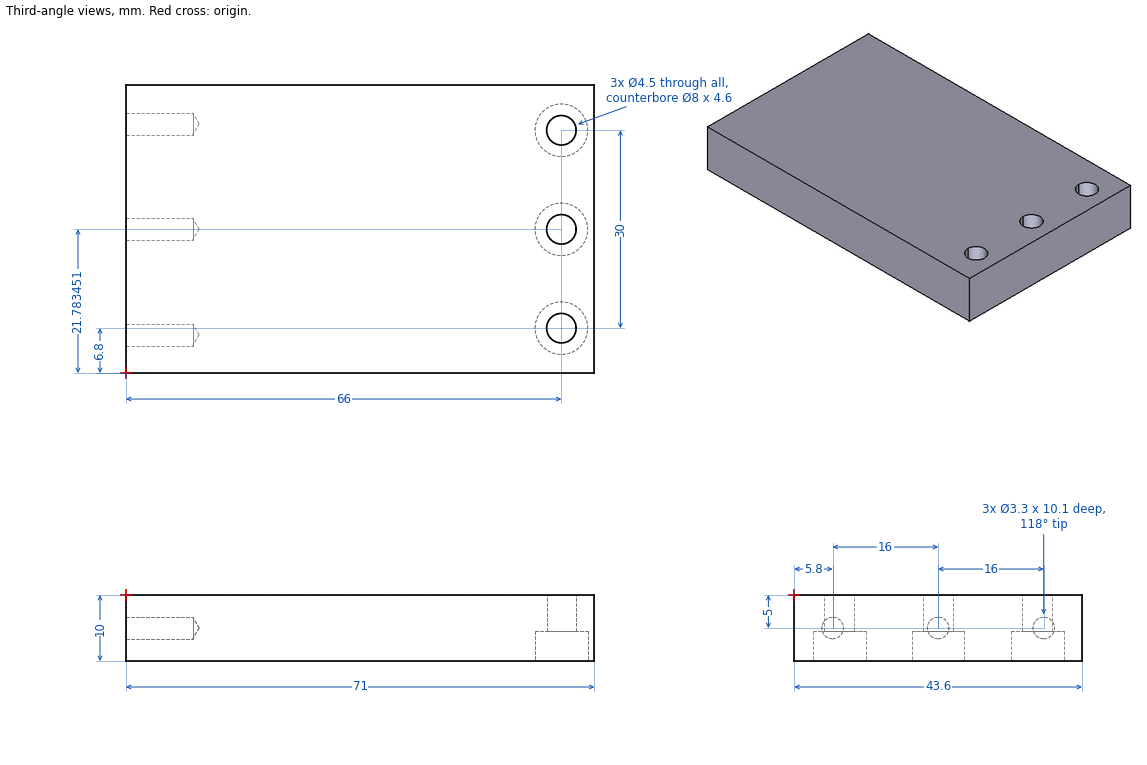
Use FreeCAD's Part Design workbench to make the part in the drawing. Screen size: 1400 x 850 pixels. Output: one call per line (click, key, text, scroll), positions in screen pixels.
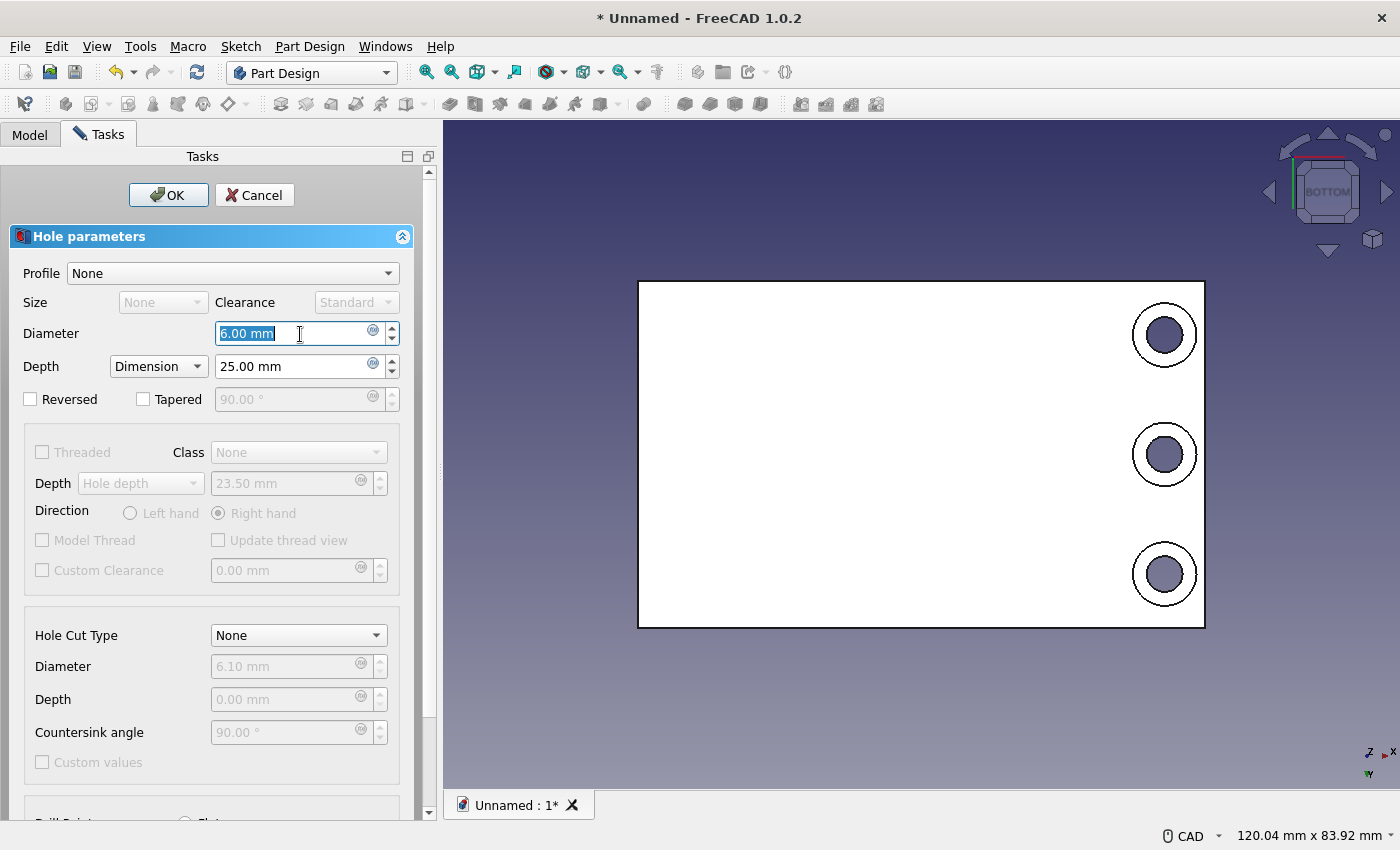
text(3.3)
key(Tab)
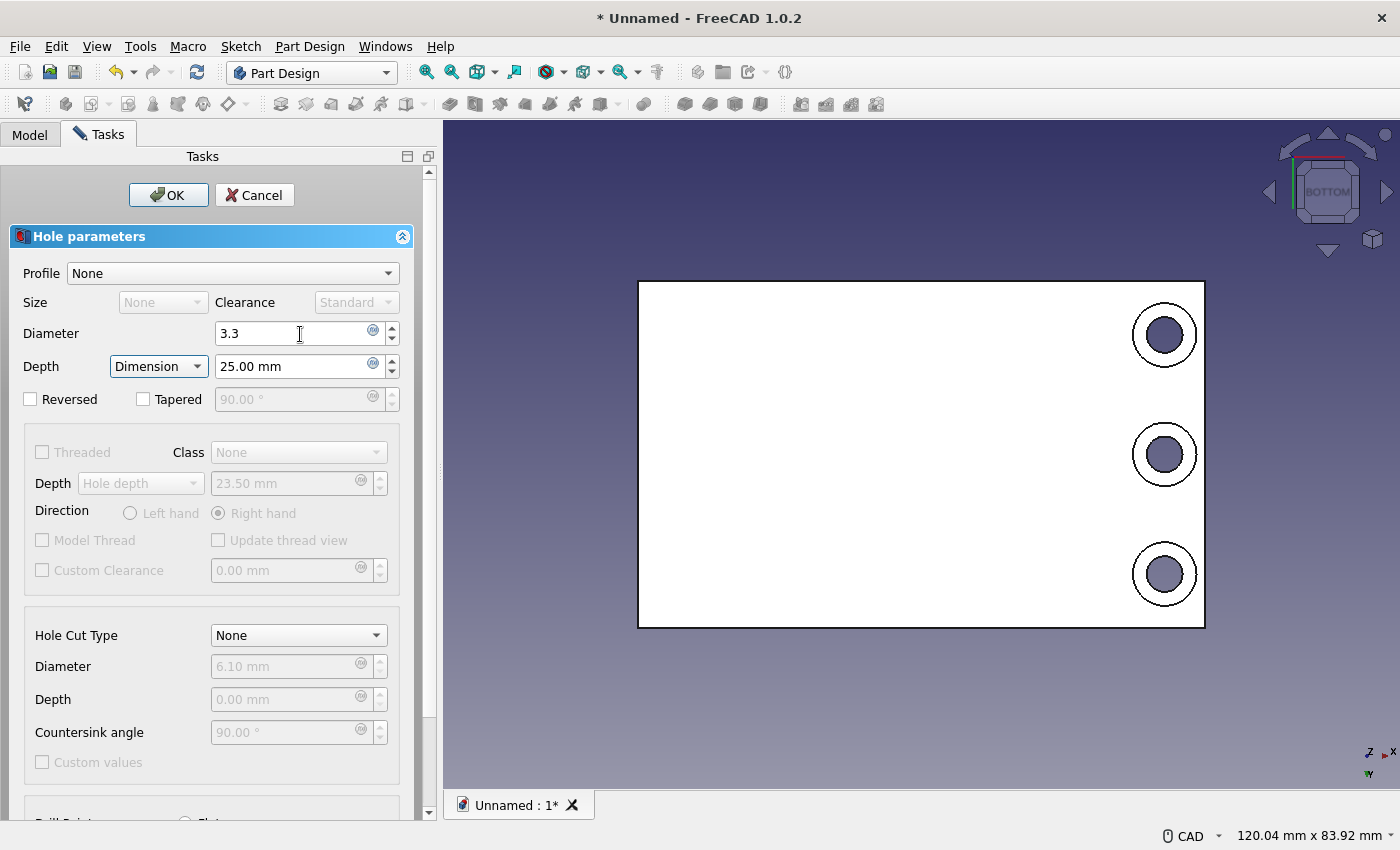
triple_click(300, 366)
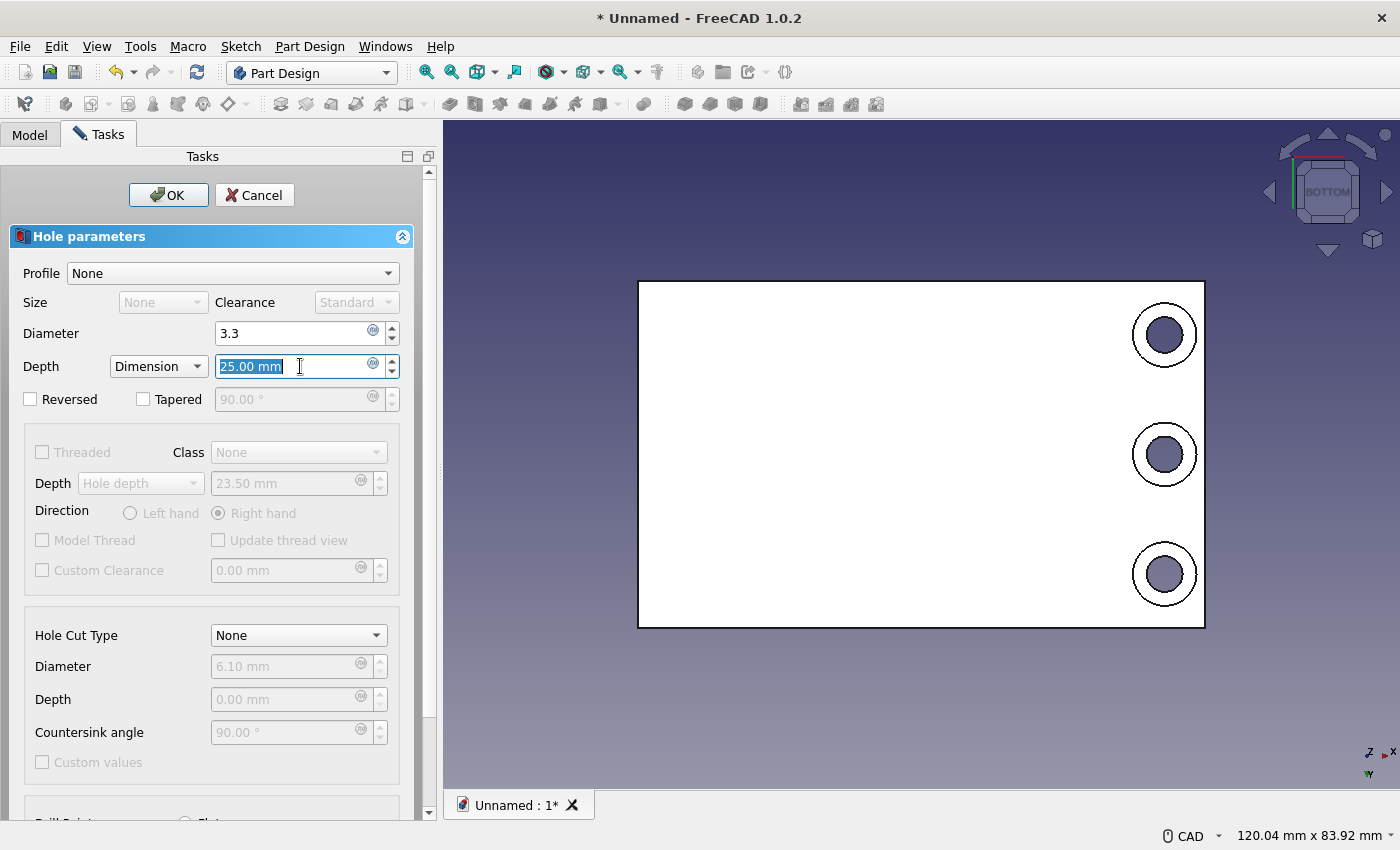
text(10.1)
key(Tab)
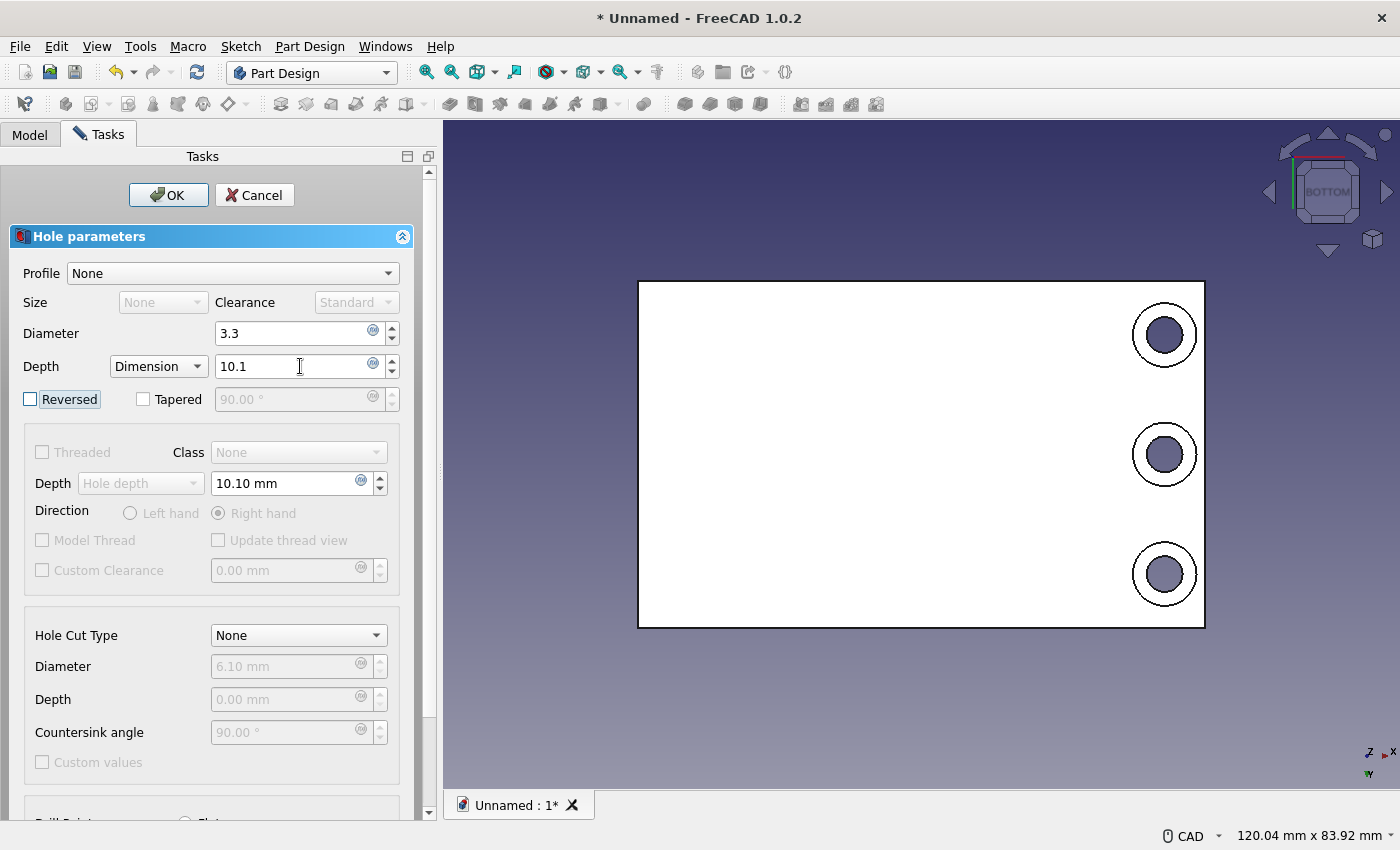
click(31, 399)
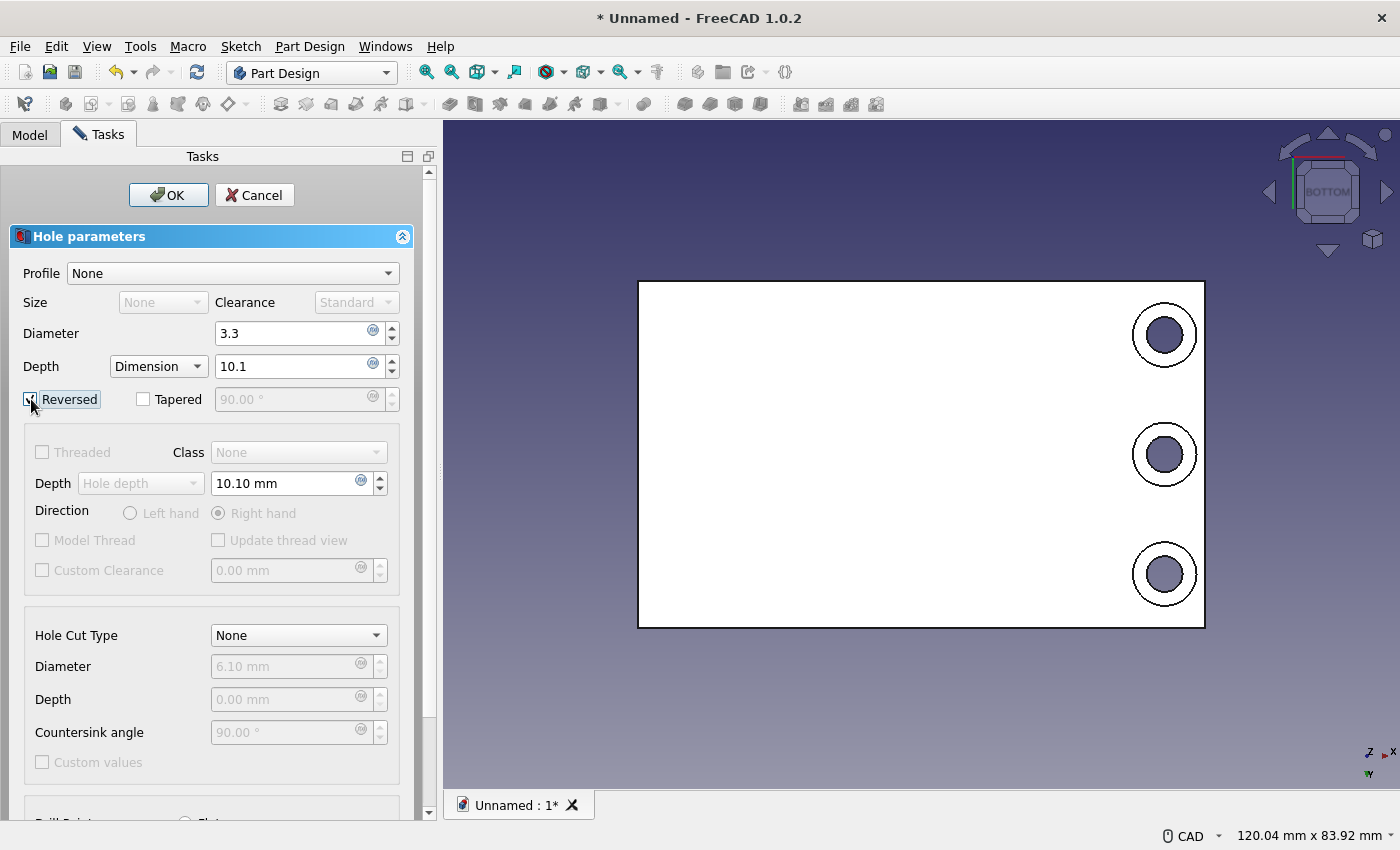
click(169, 195)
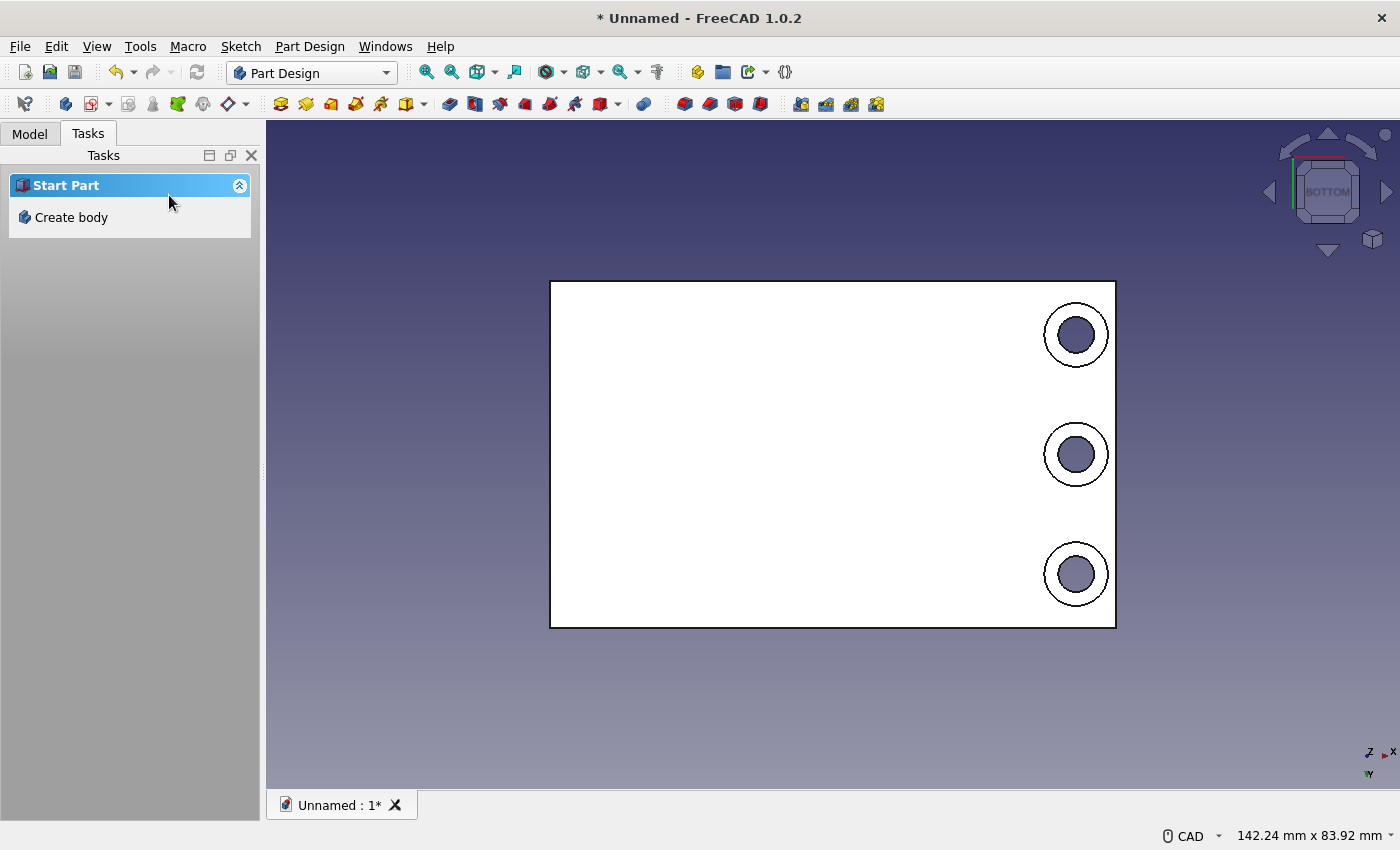
key(0)